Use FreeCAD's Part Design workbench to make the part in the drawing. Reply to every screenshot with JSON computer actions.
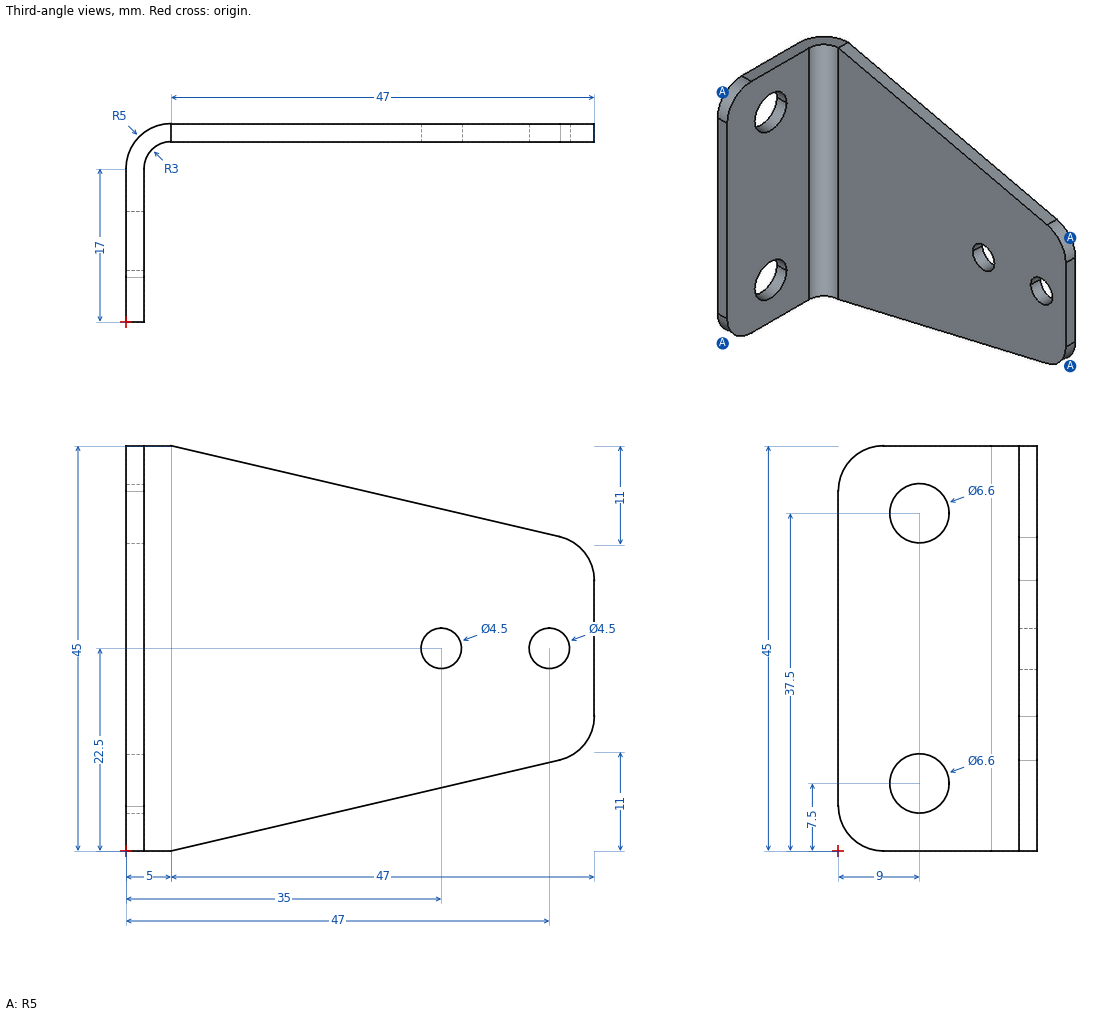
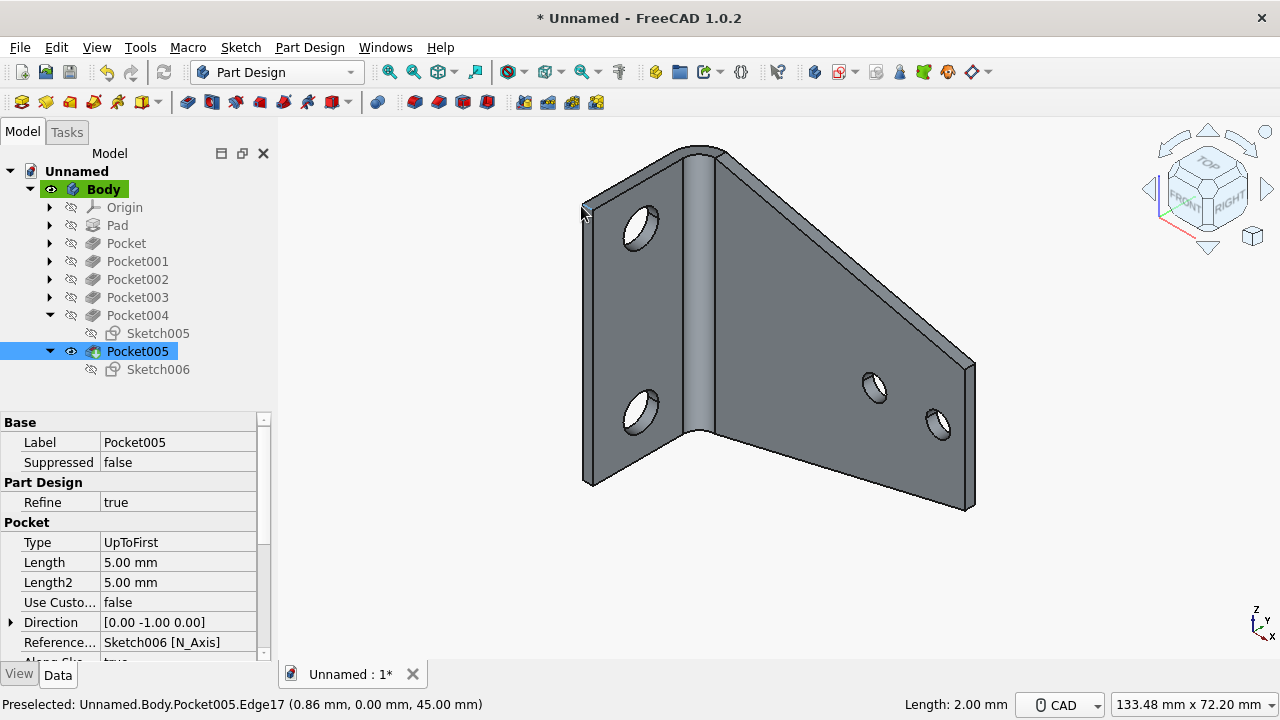
{"action": "left_click", "coordinate": [971, 365], "text": "ctrl"}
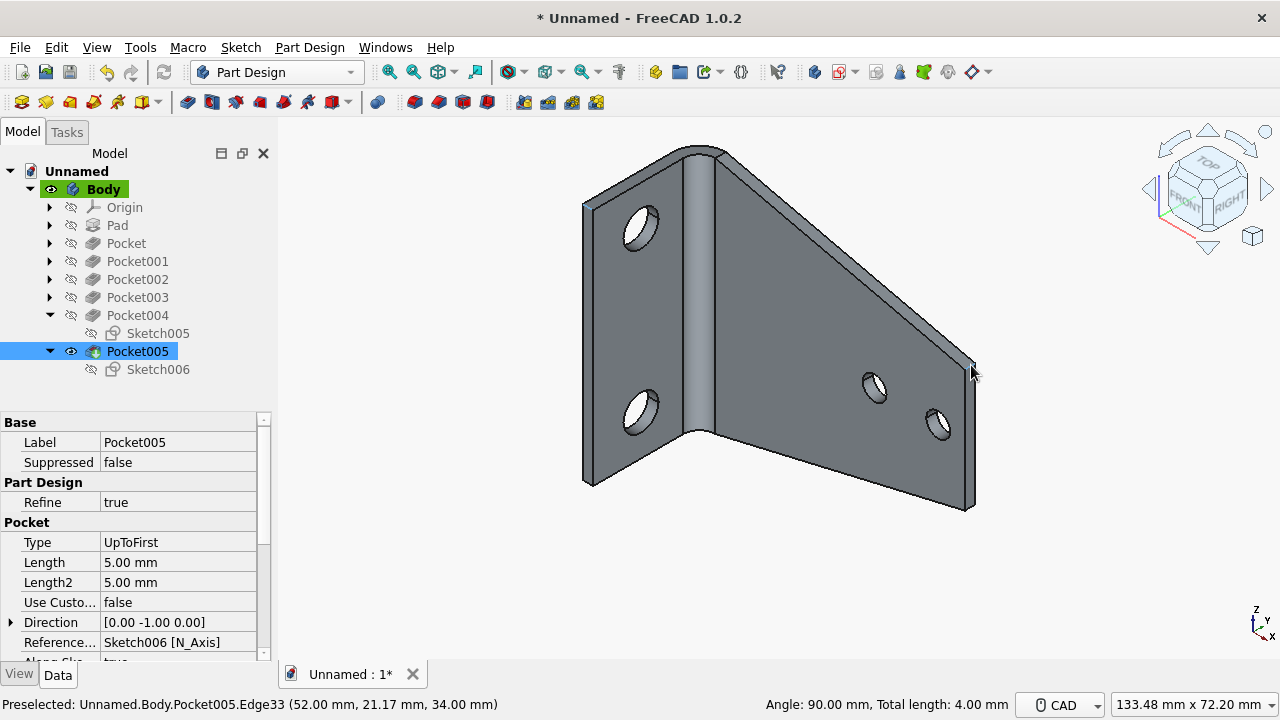
{"action": "scroll", "coordinate": [588, 482], "scroll_direction": "up", "scroll_amount": 5}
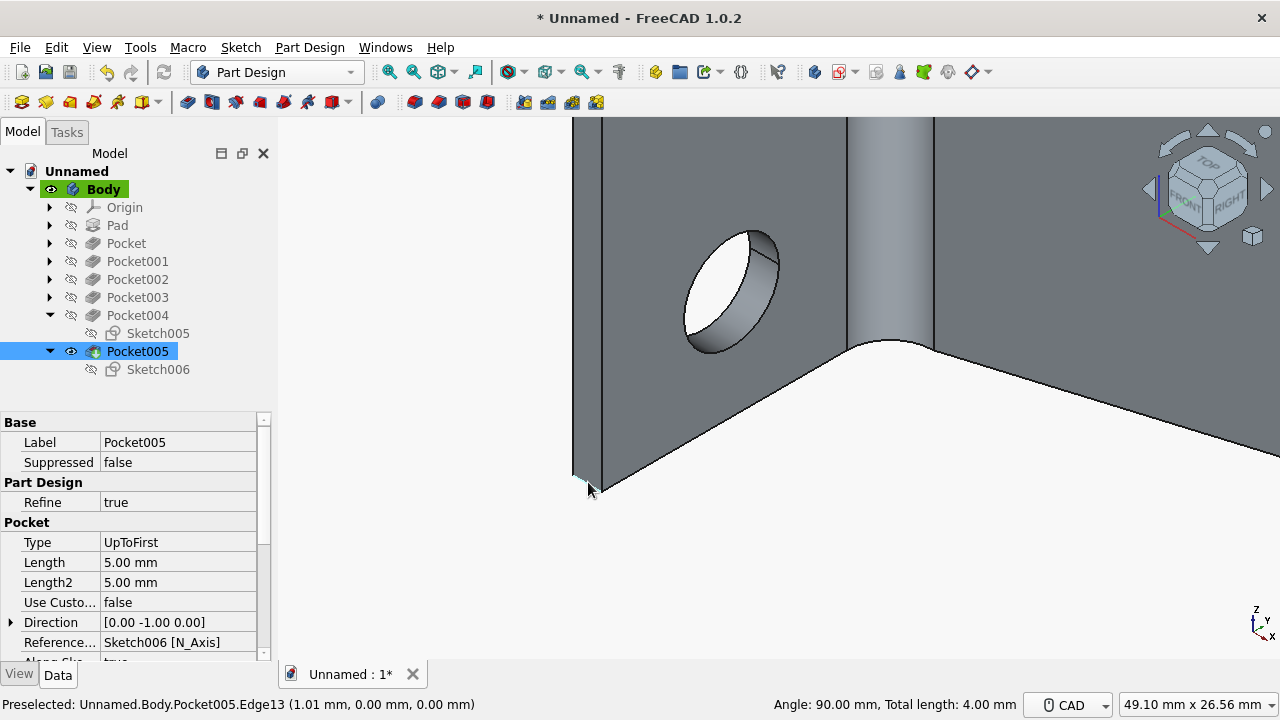
{"action": "key", "text": "v f"}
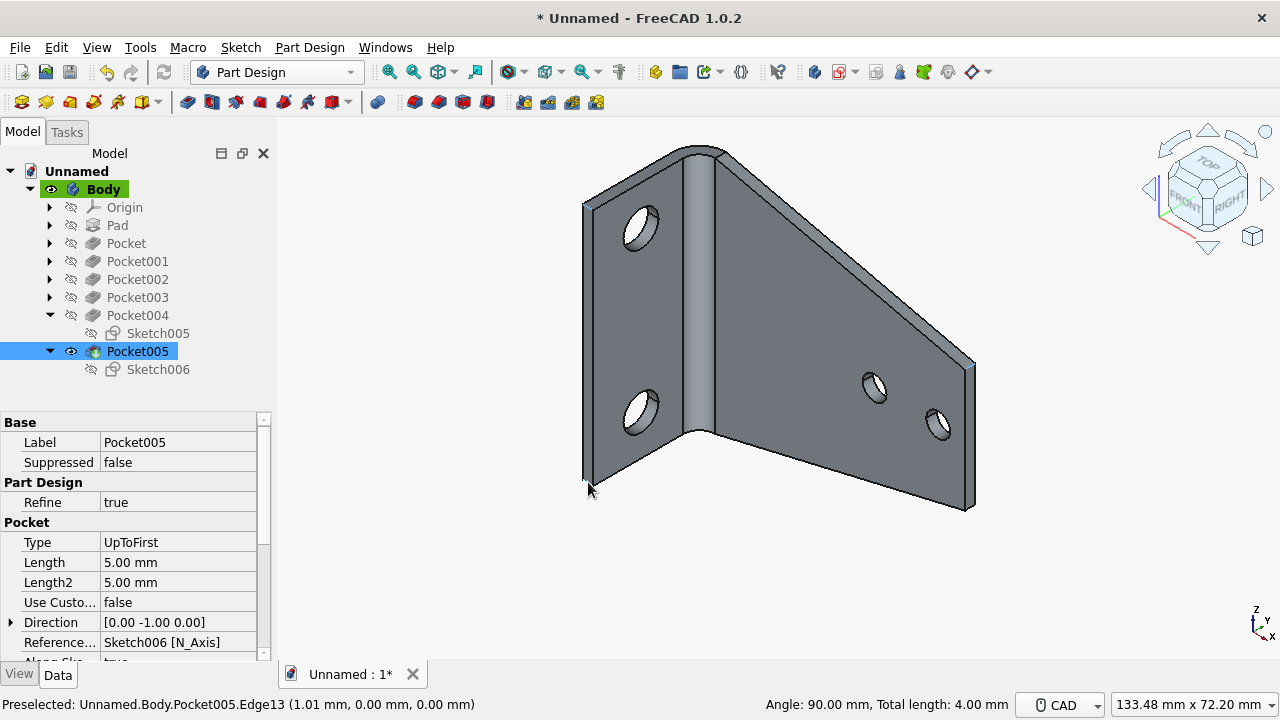
{"action": "key", "text": "2"}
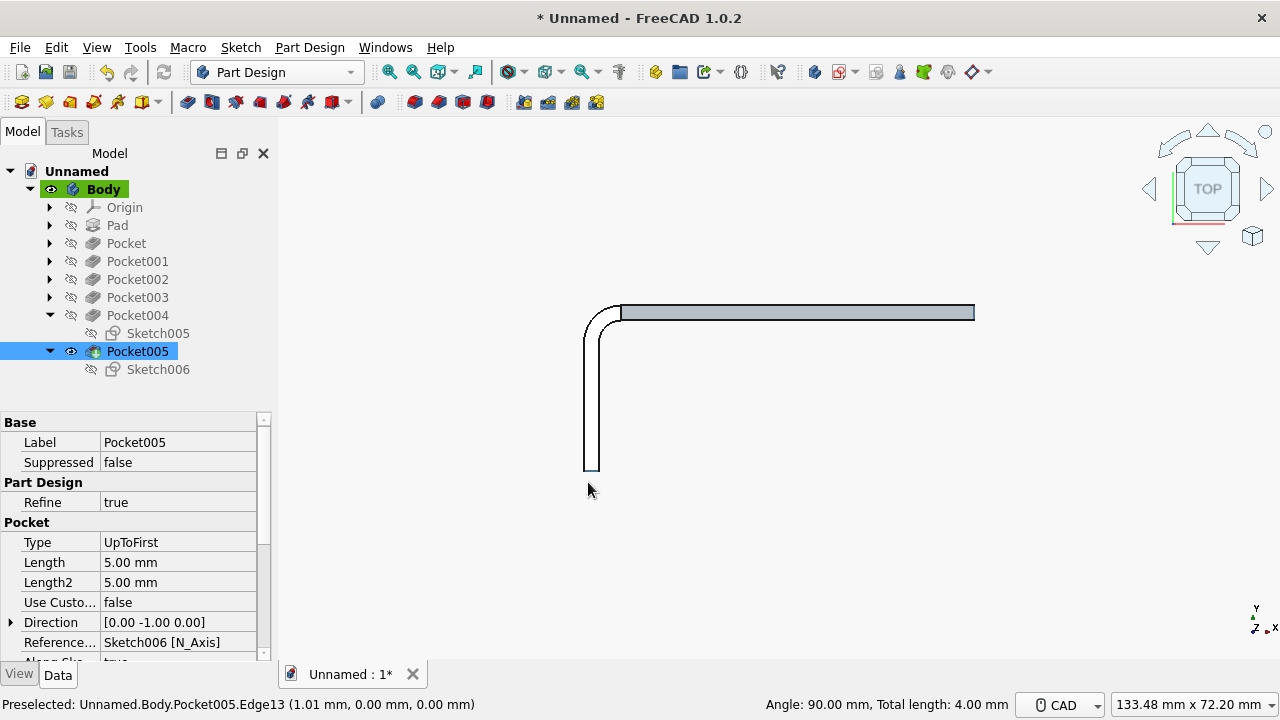
{"action": "key", "text": "v f"}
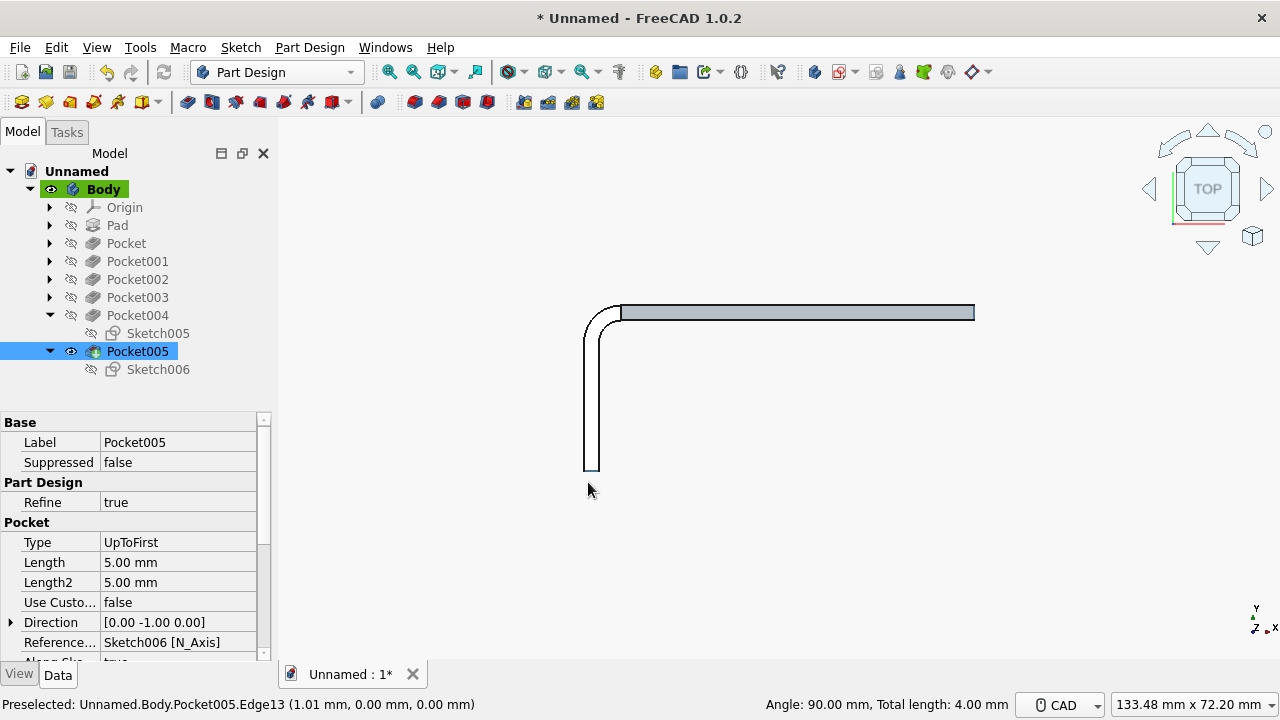
{"action": "scroll", "coordinate": [591, 470], "scroll_direction": "up", "scroll_amount": 5}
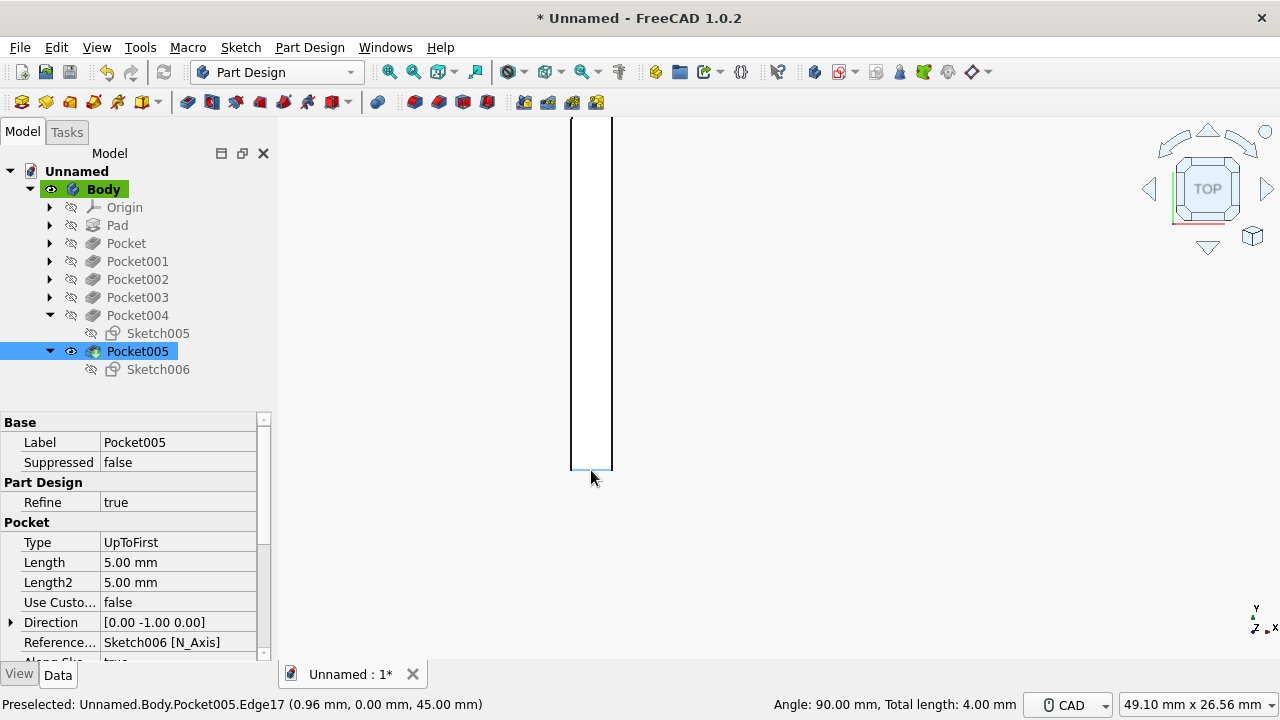
{"action": "key", "text": "v f"}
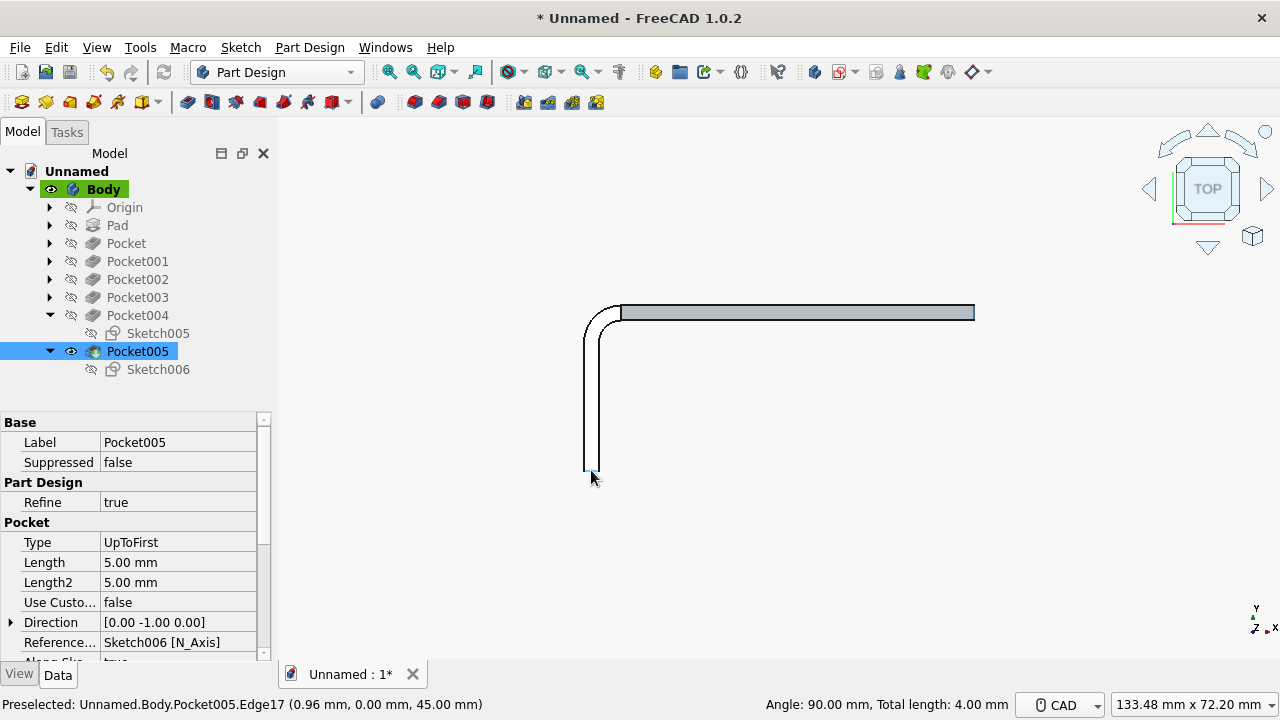
{"action": "key", "text": "1"}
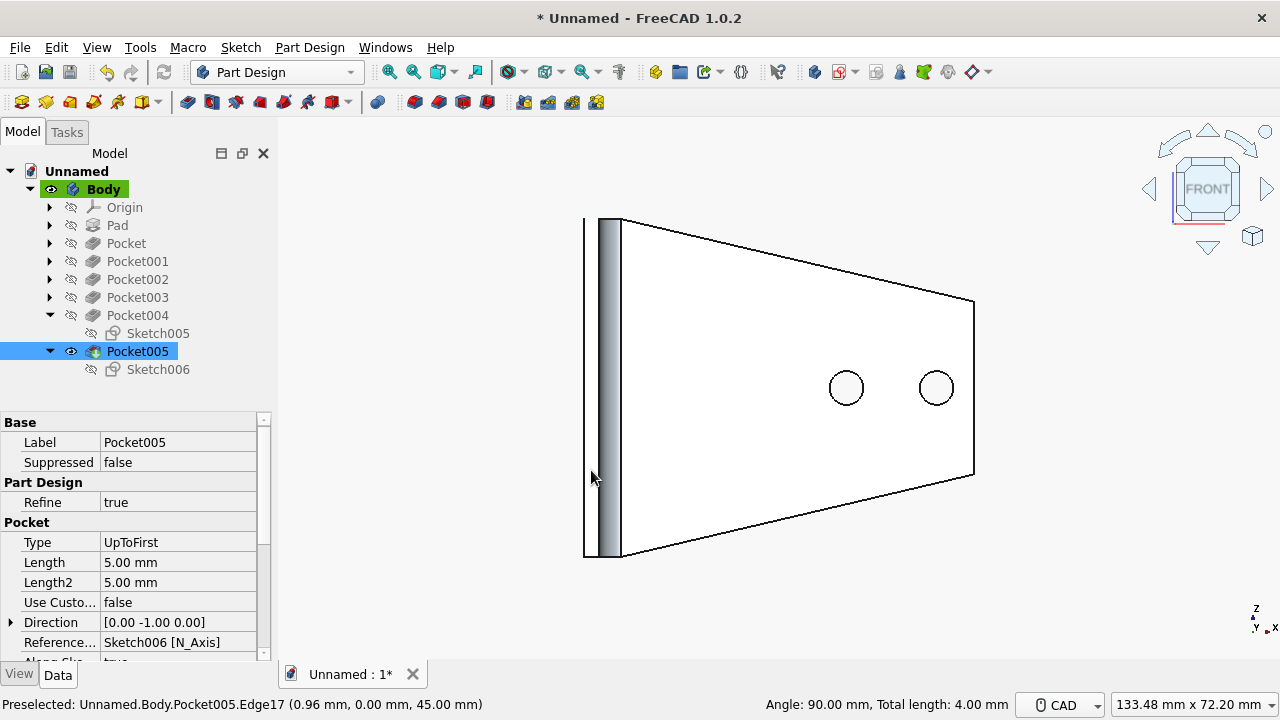
{"action": "left_click", "coordinate": [591, 556], "text": "ctrl"}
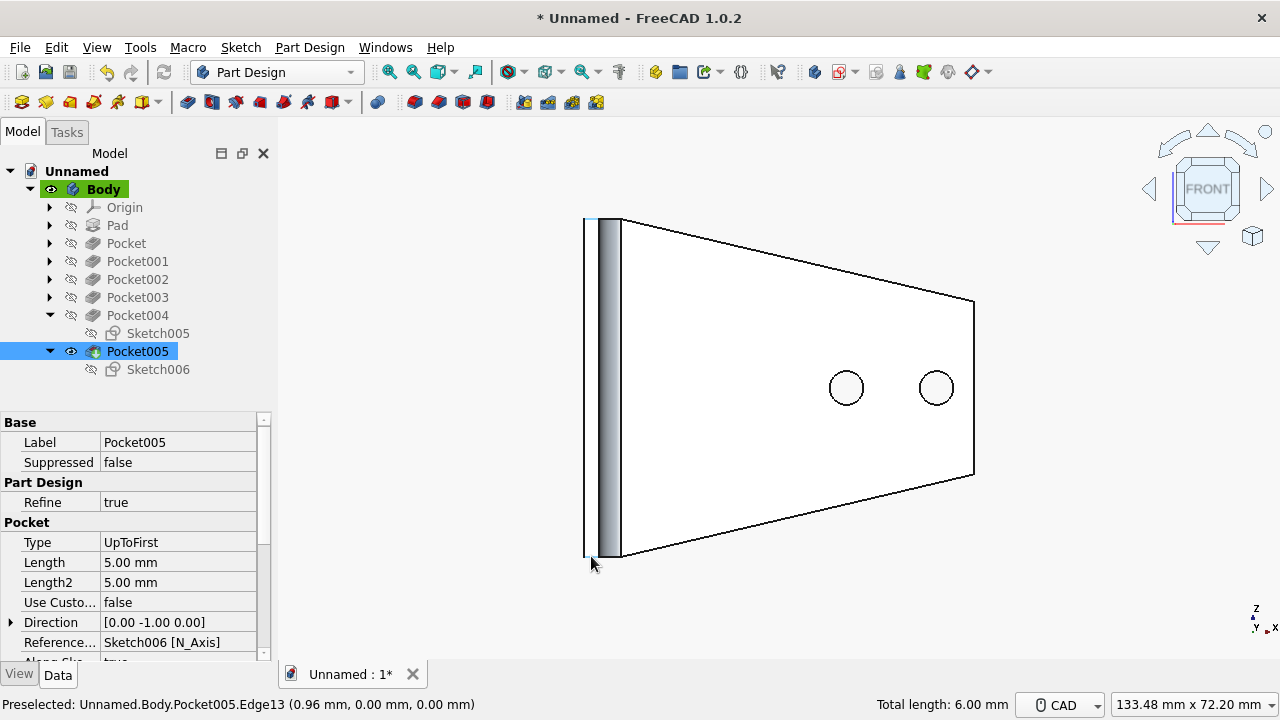
{"action": "scroll", "coordinate": [974, 473], "scroll_direction": "up", "scroll_amount": 5}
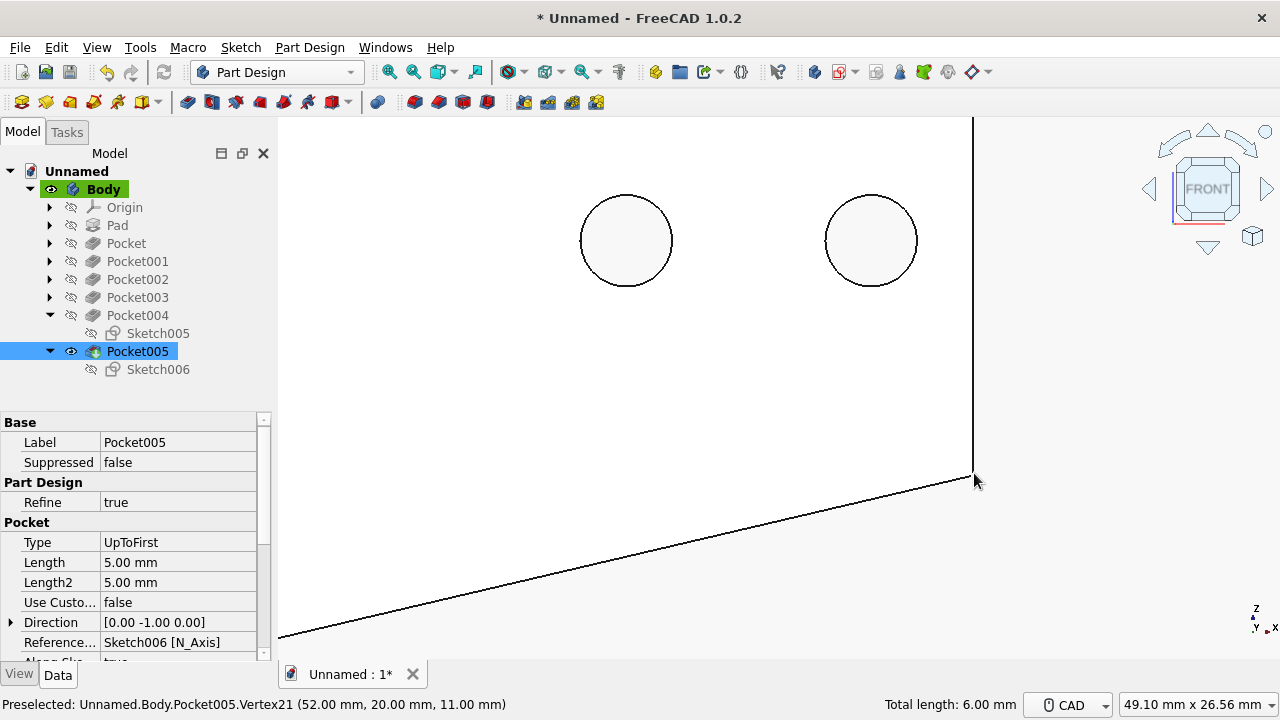
{"action": "key", "text": "v f"}